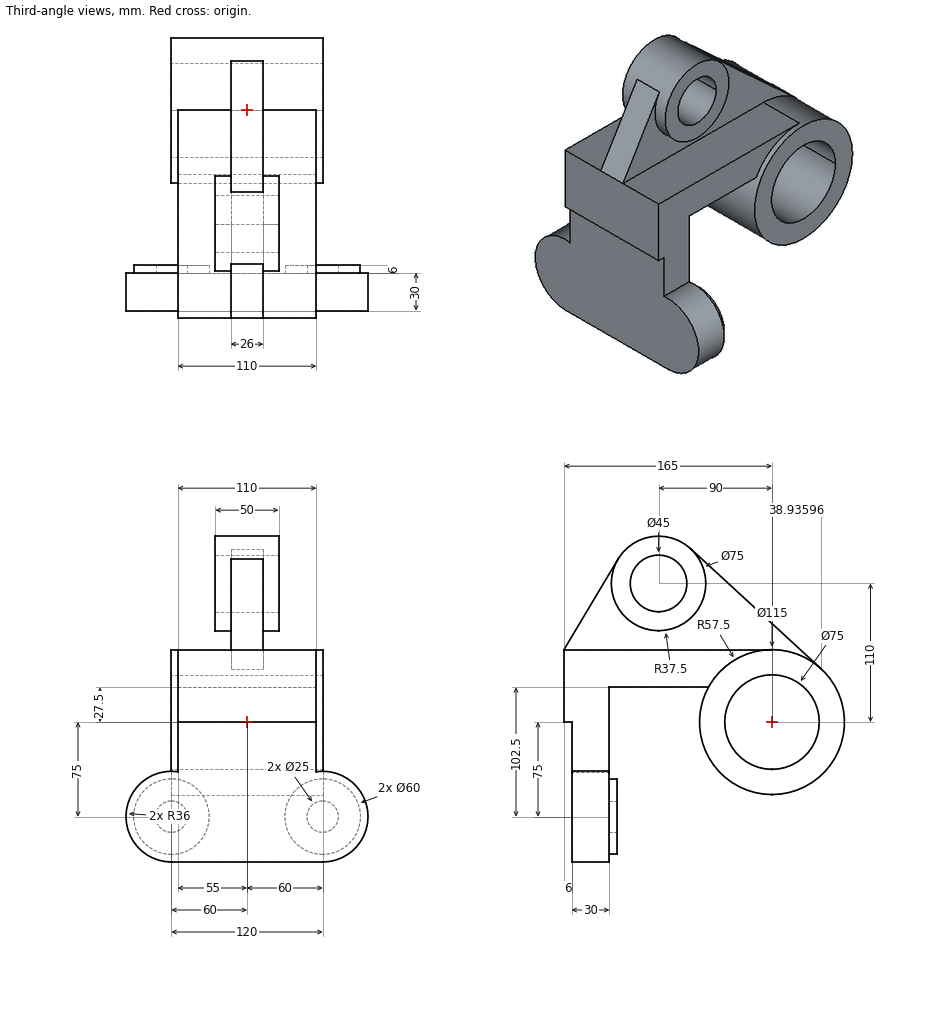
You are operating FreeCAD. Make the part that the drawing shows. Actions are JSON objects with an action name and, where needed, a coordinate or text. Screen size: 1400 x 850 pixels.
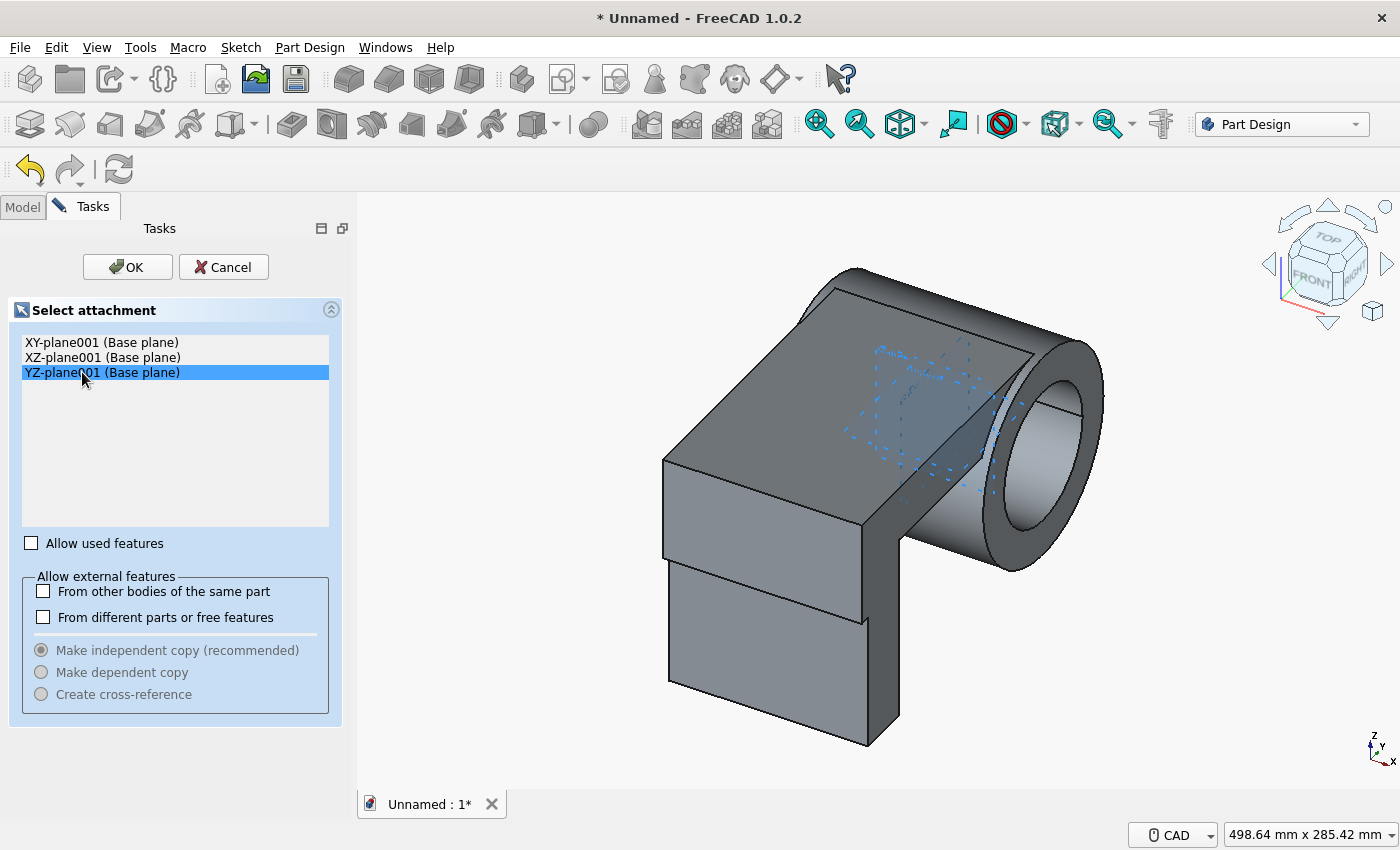
{"action": "left_click", "coordinate": [128, 267]}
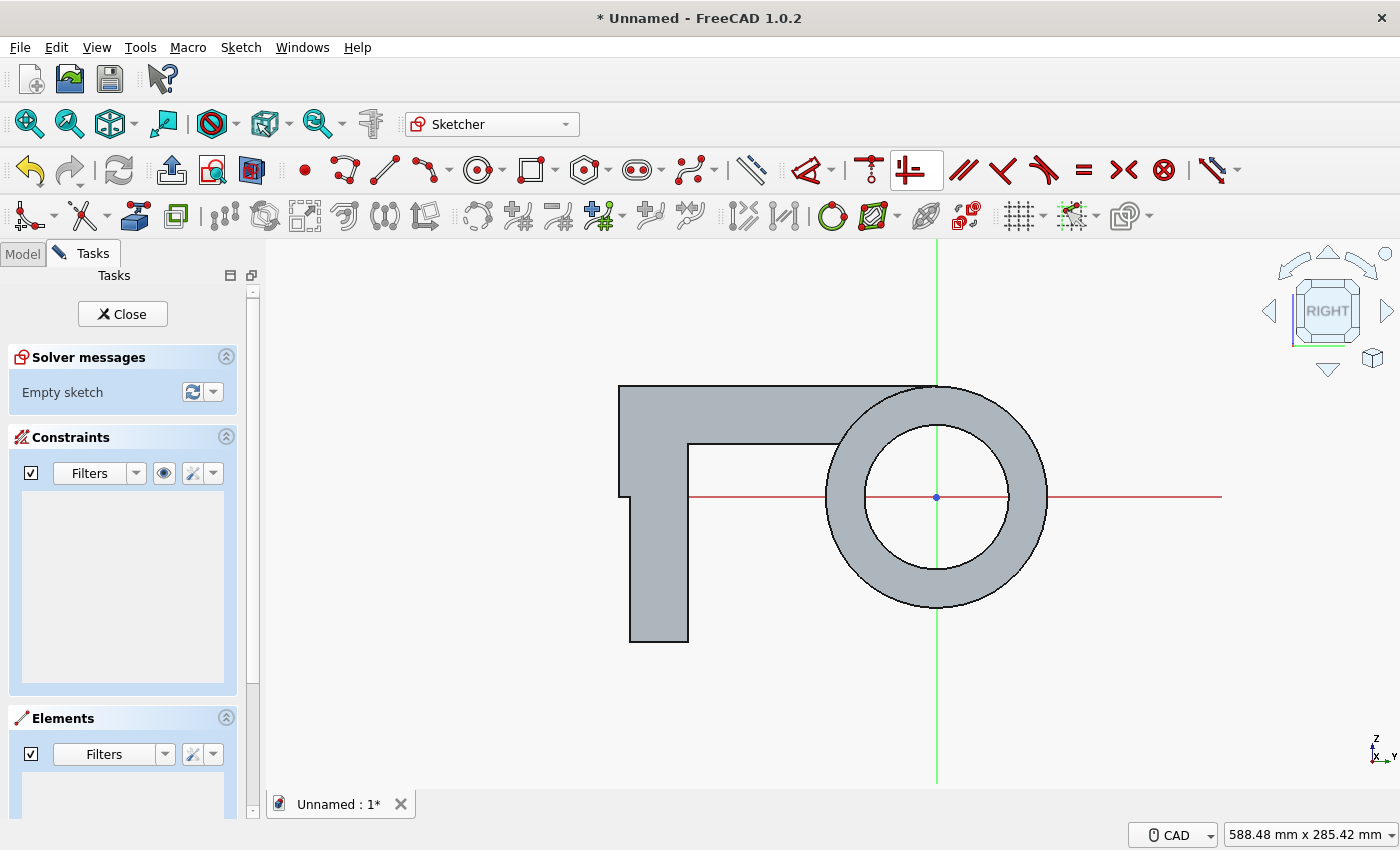
{"action": "scroll", "coordinate": [542, 761], "scroll_direction": "down", "scroll_amount": 1}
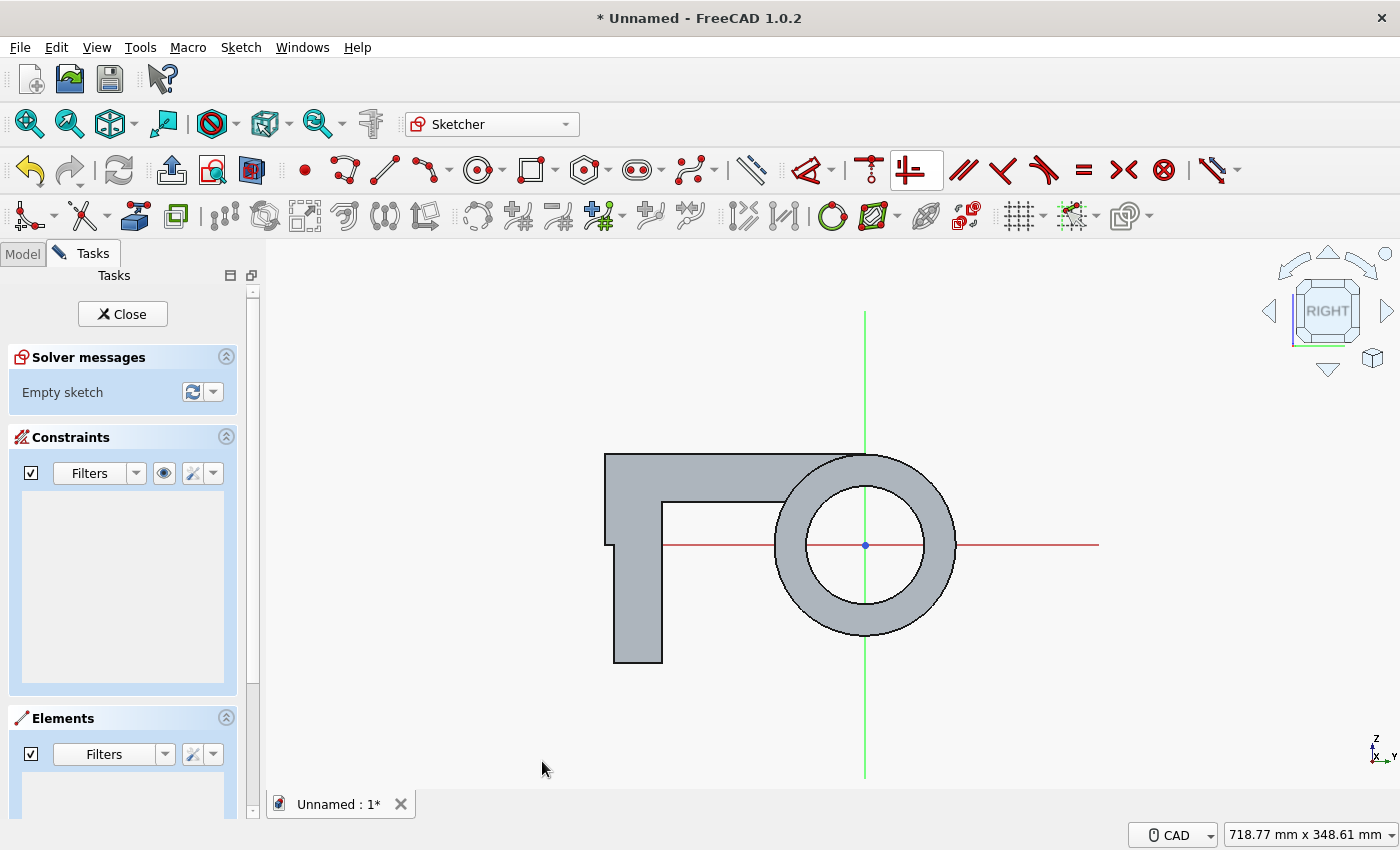
{"action": "scroll", "coordinate": [765, 267], "scroll_direction": "up", "scroll_amount": 2}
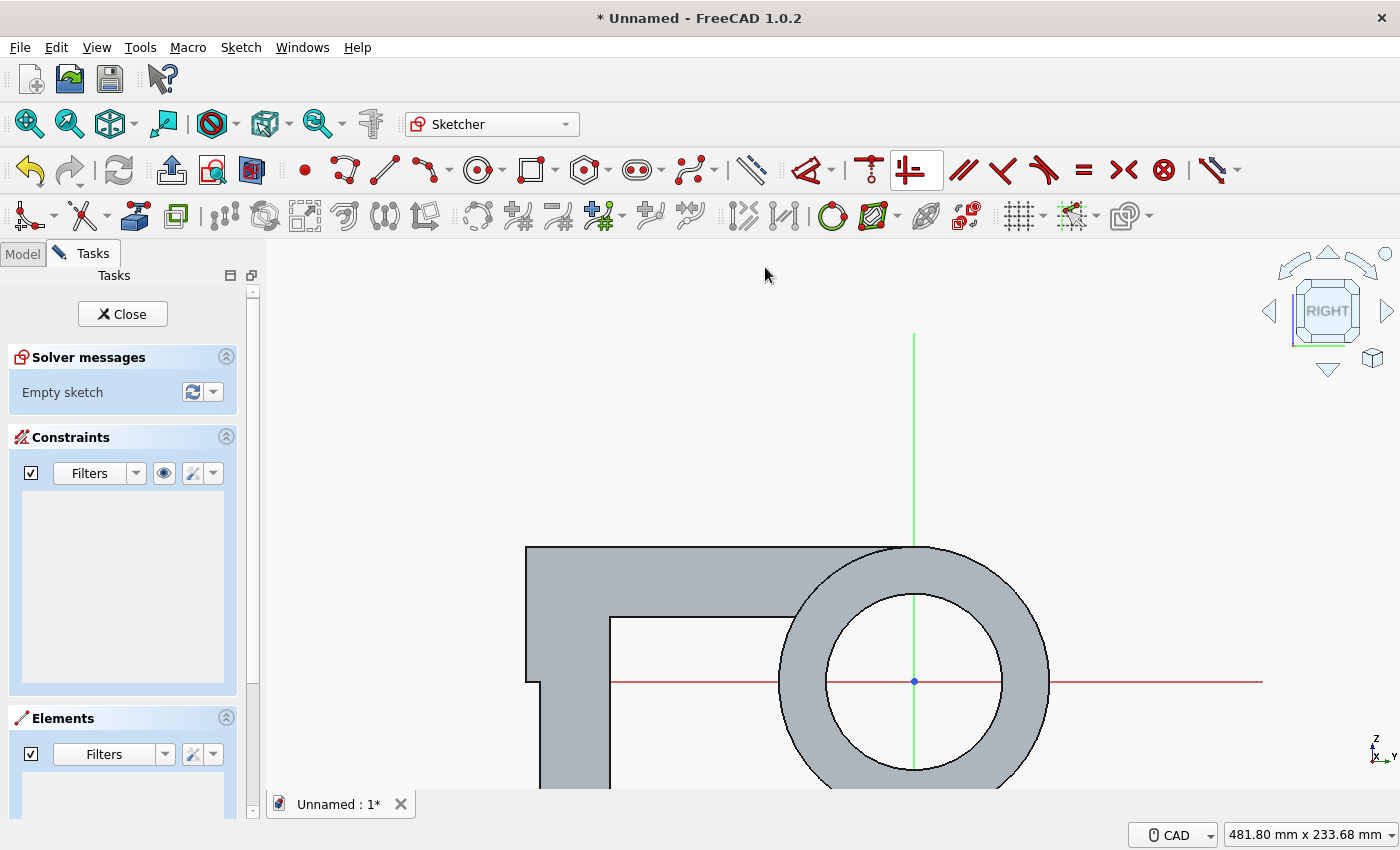
{"action": "left_click", "coordinate": [478, 170]}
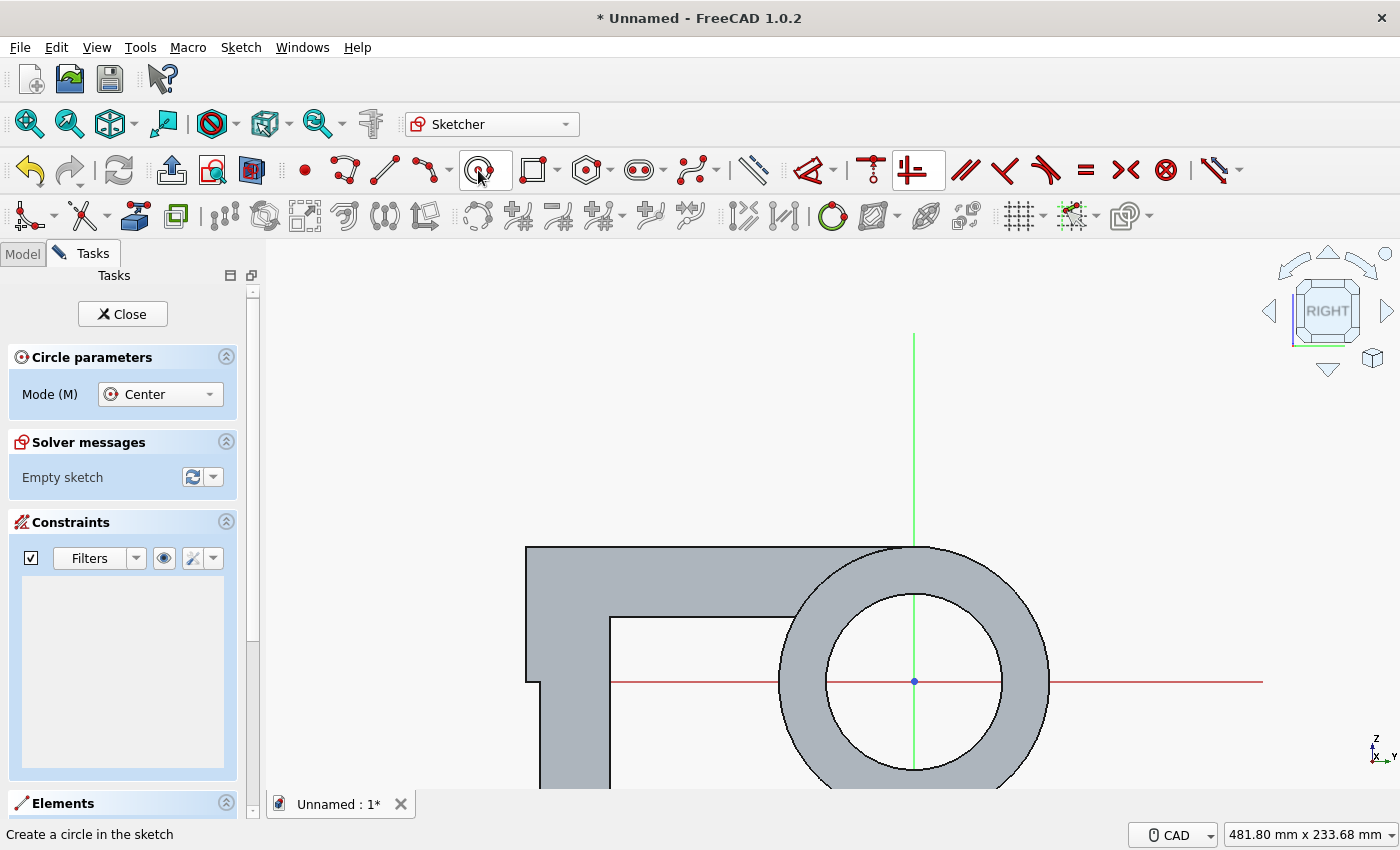
{"action": "left_click", "coordinate": [702, 423]}
{"action": "mouse_move", "coordinate": [765, 361]}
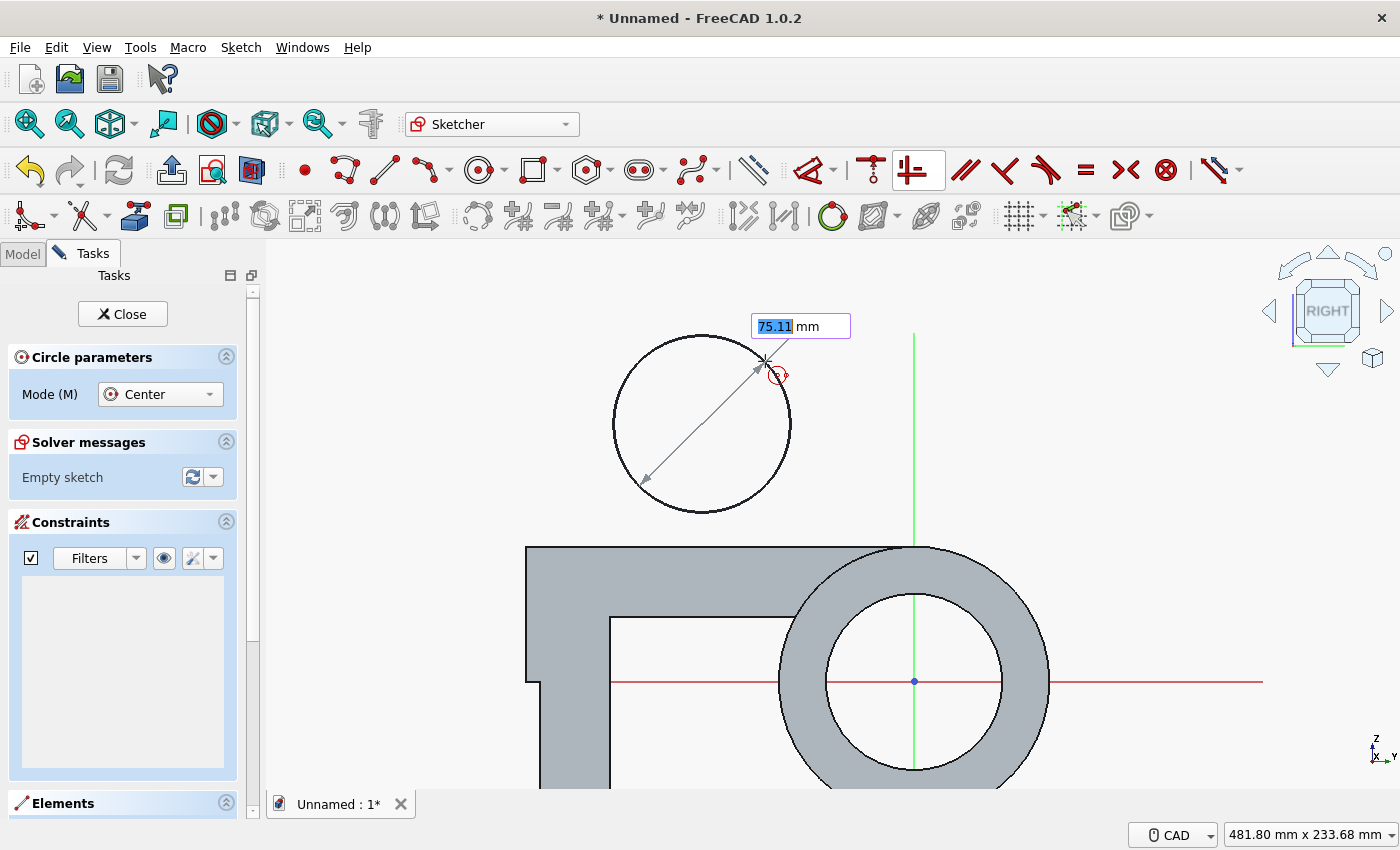
{"action": "type", "text": "75"}
{"action": "key", "text": "Return"}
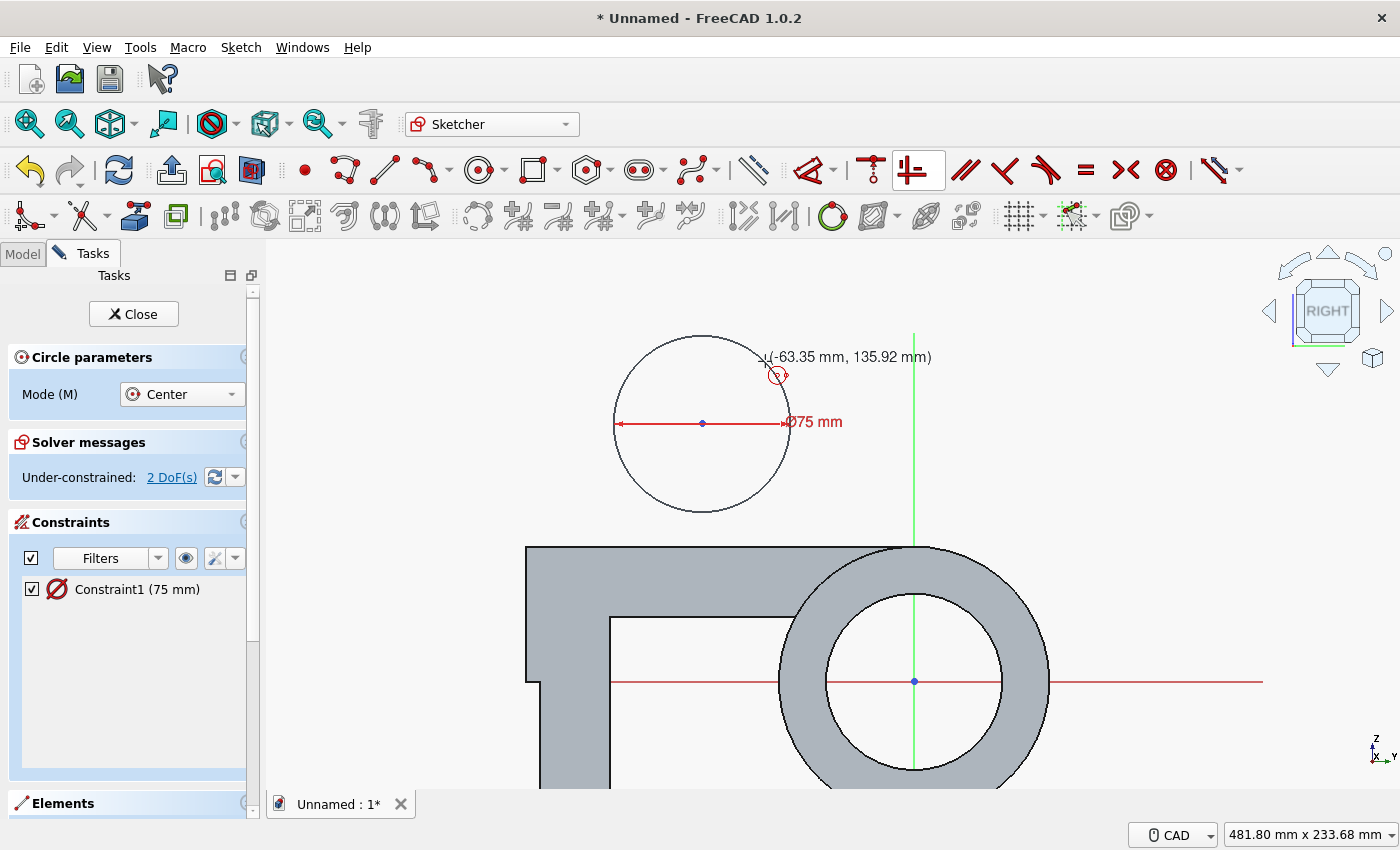
{"action": "left_click", "coordinate": [702, 424]}
{"action": "mouse_move", "coordinate": [740, 386]}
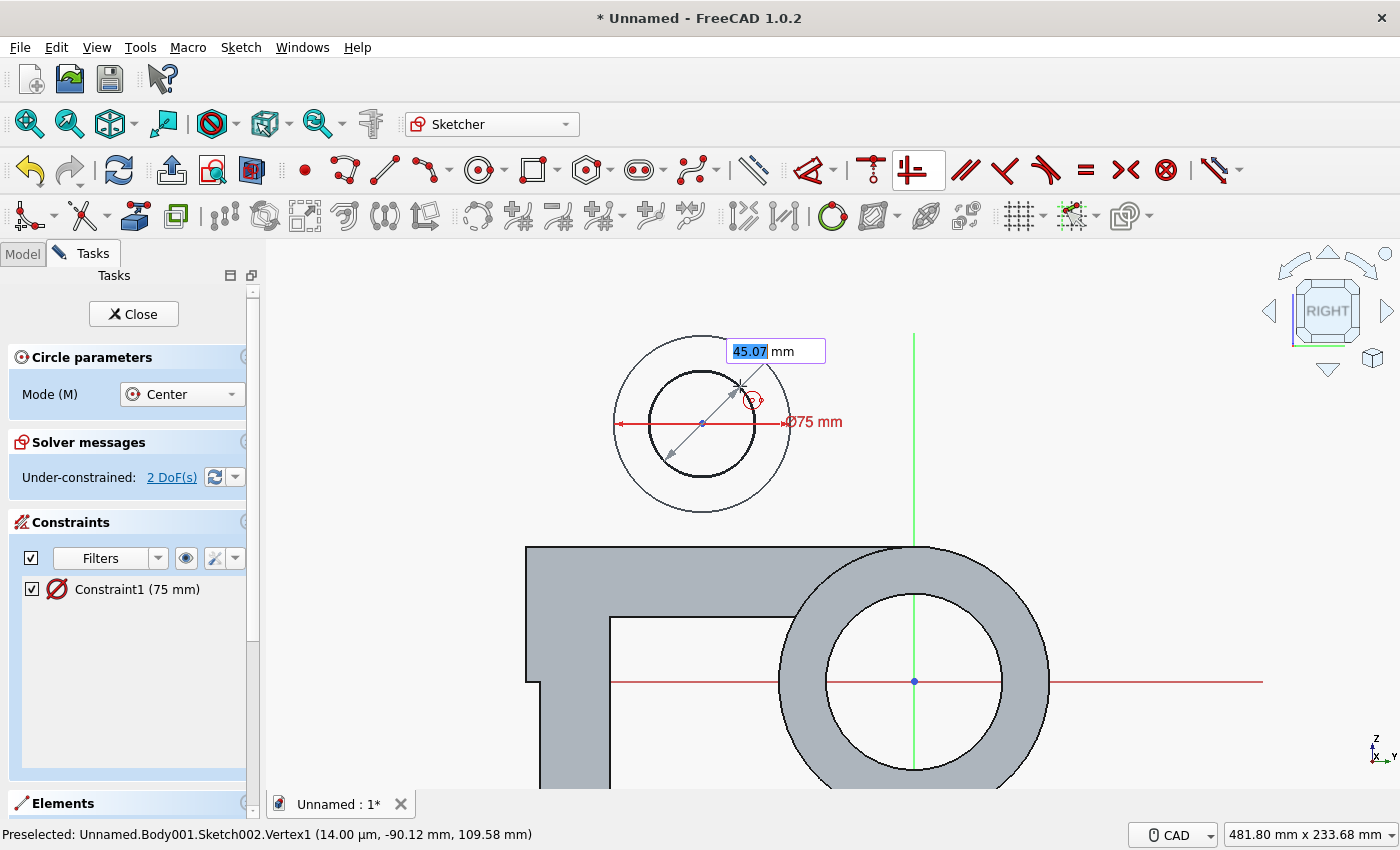
{"action": "type", "text": "45"}
{"action": "key", "text": "Return"}
{"action": "key", "text": "Escape"}